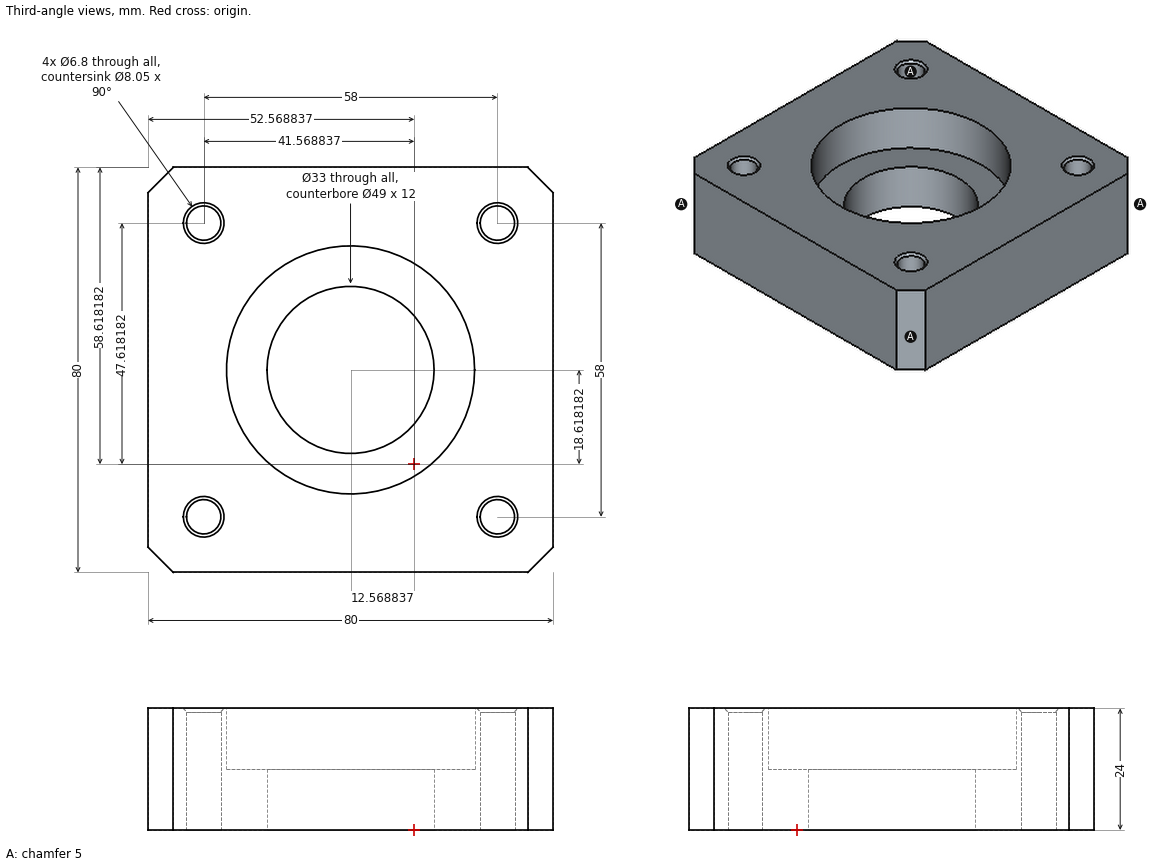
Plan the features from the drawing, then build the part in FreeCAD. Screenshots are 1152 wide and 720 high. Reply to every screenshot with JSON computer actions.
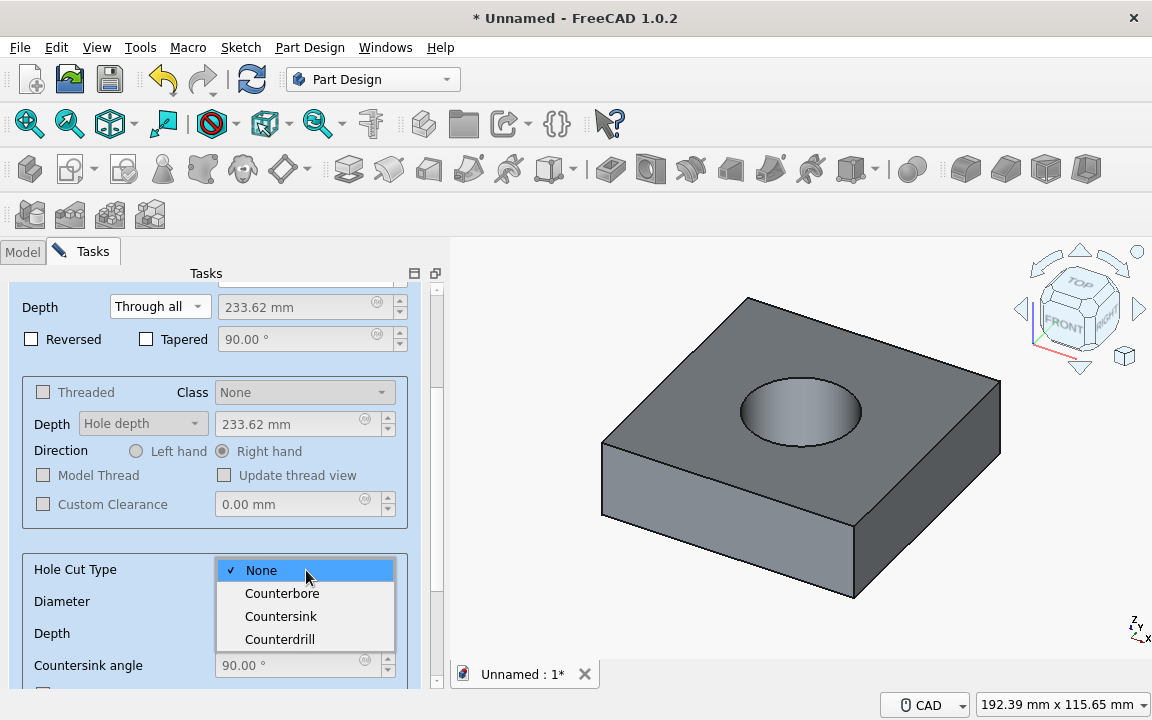
{"action": "left_click", "coordinate": [304, 594]}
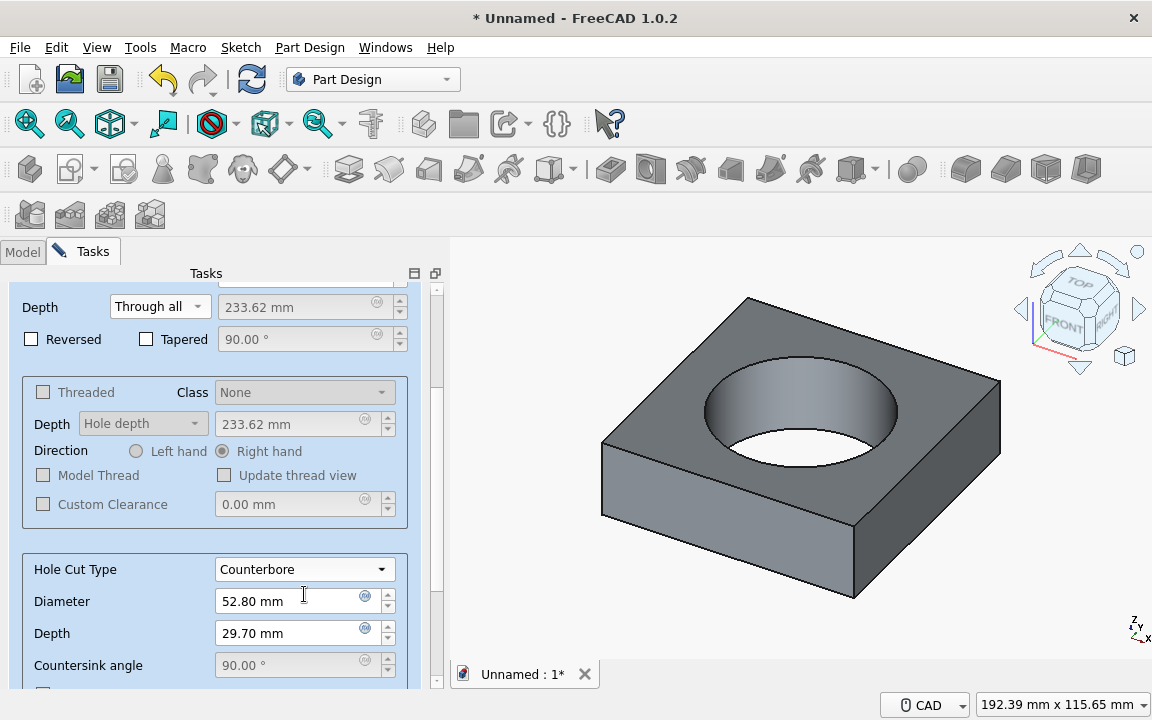
{"action": "triple_click", "coordinate": [298, 601]}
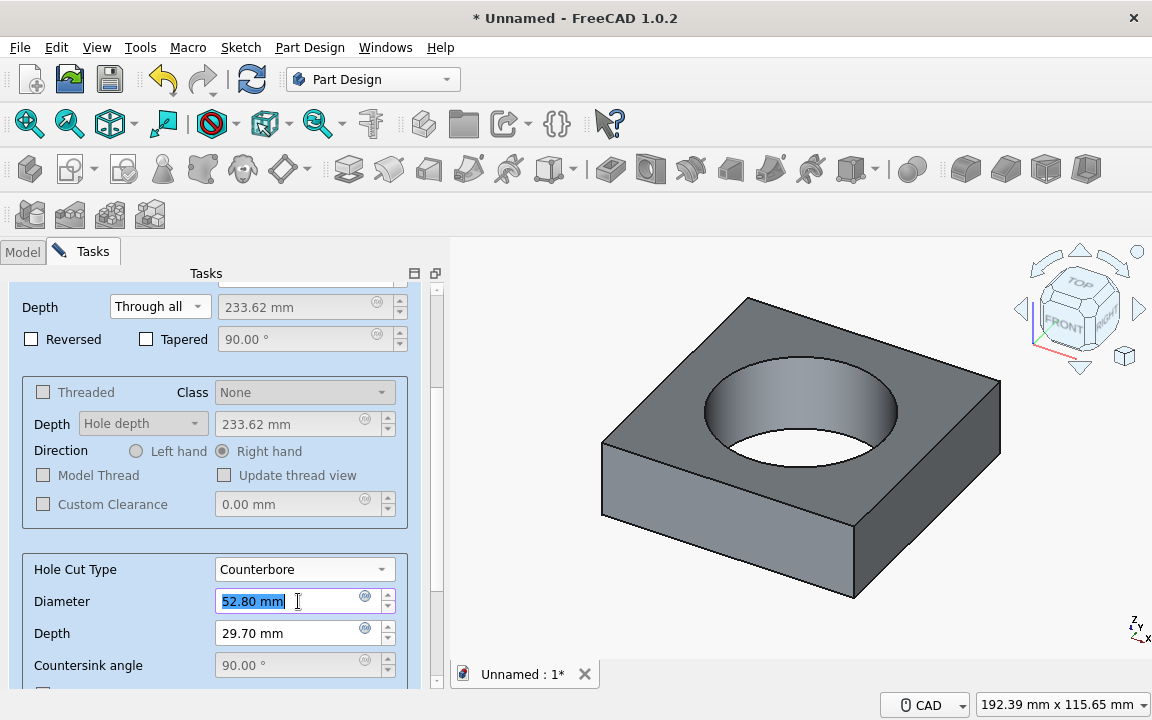
{"action": "type", "text": "49"}
{"action": "key", "text": "Tab"}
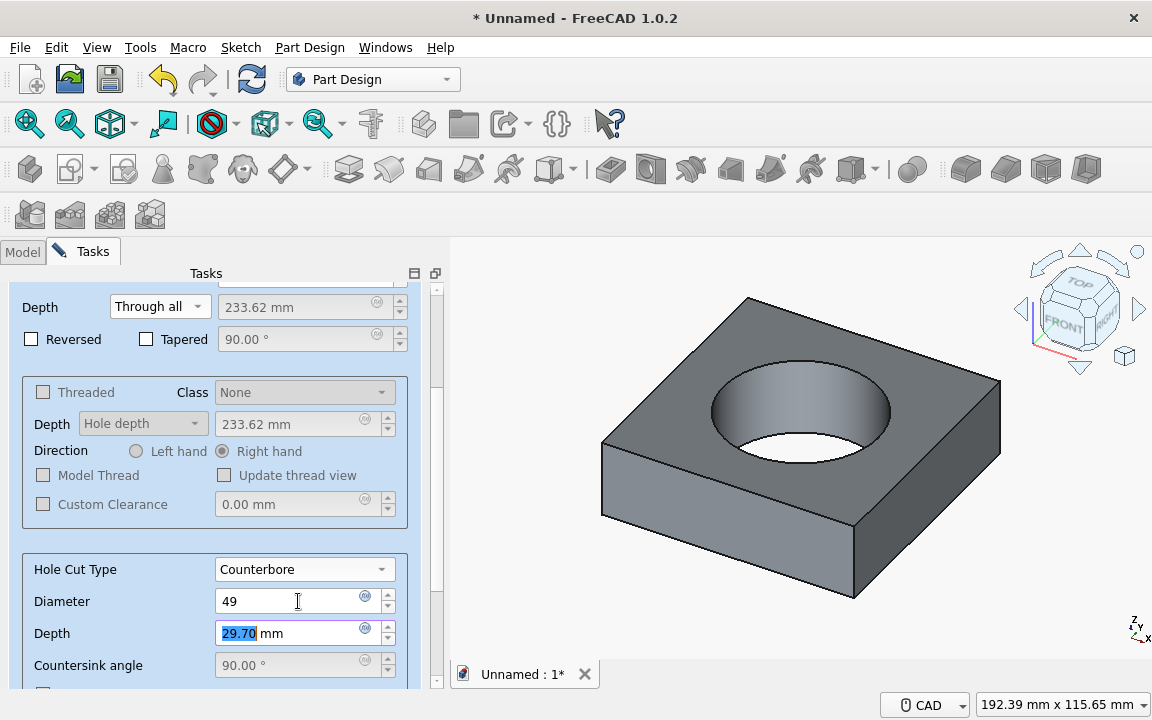
{"action": "type", "text": "12"}
{"action": "key", "text": "Tab"}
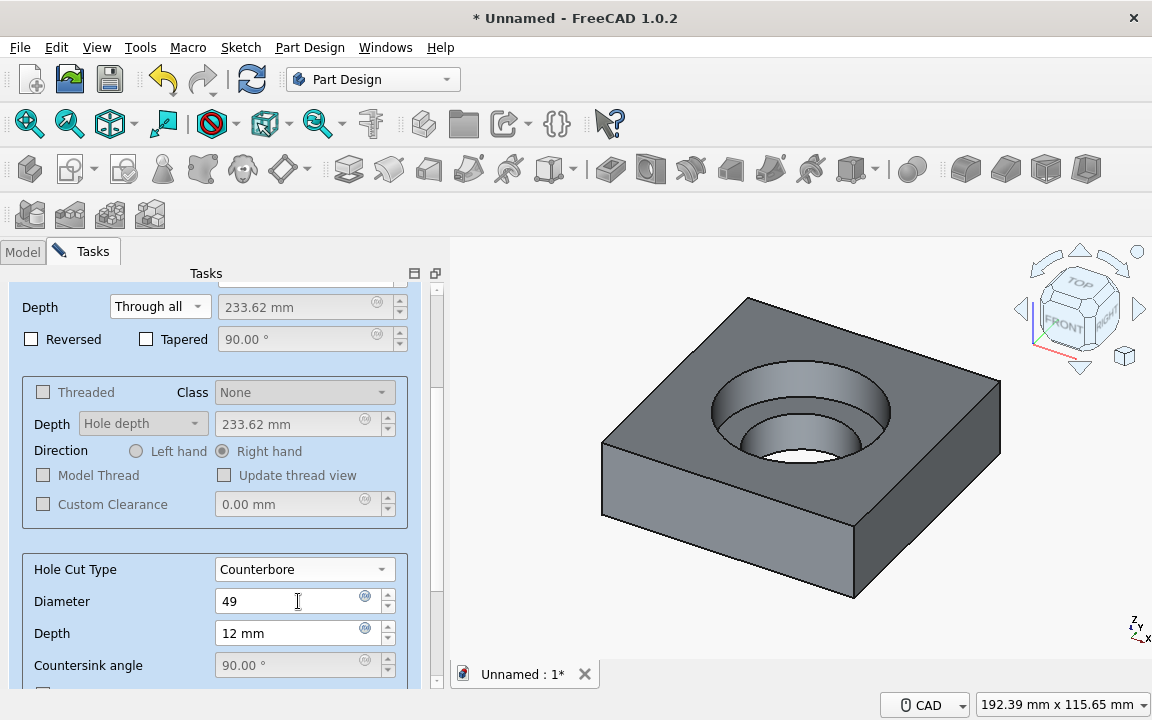
{"action": "scroll", "coordinate": [437, 486], "scroll_direction": "up", "scroll_amount": 4}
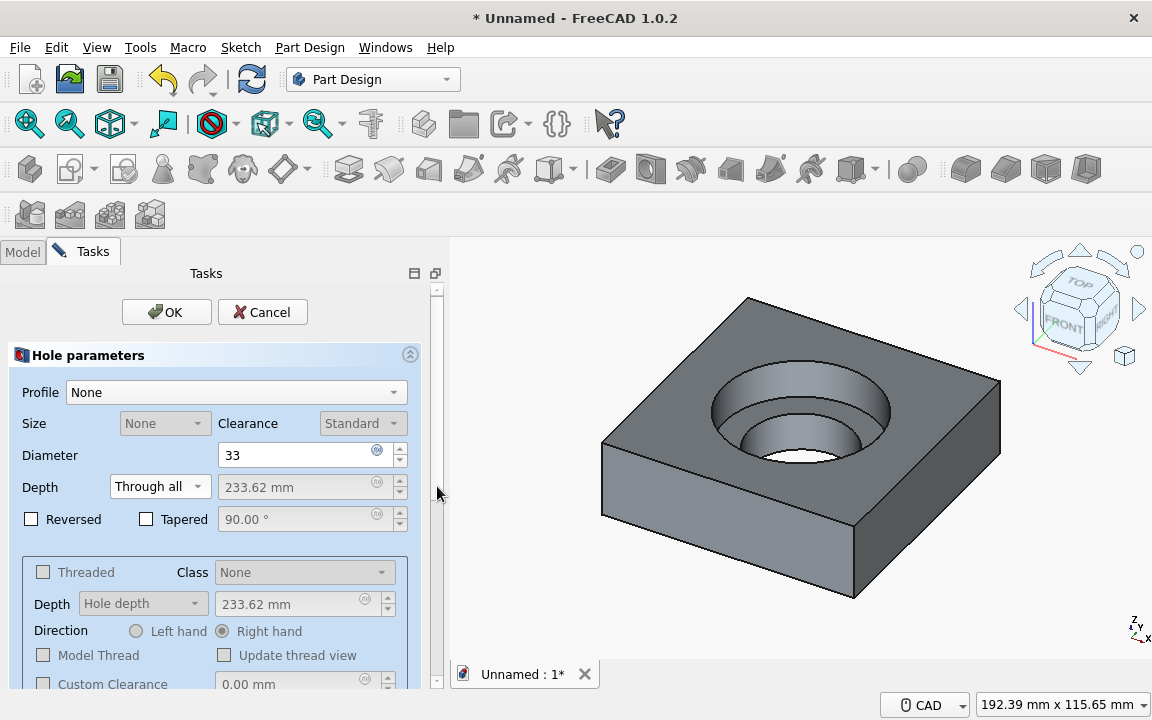
{"action": "left_click", "coordinate": [167, 312]}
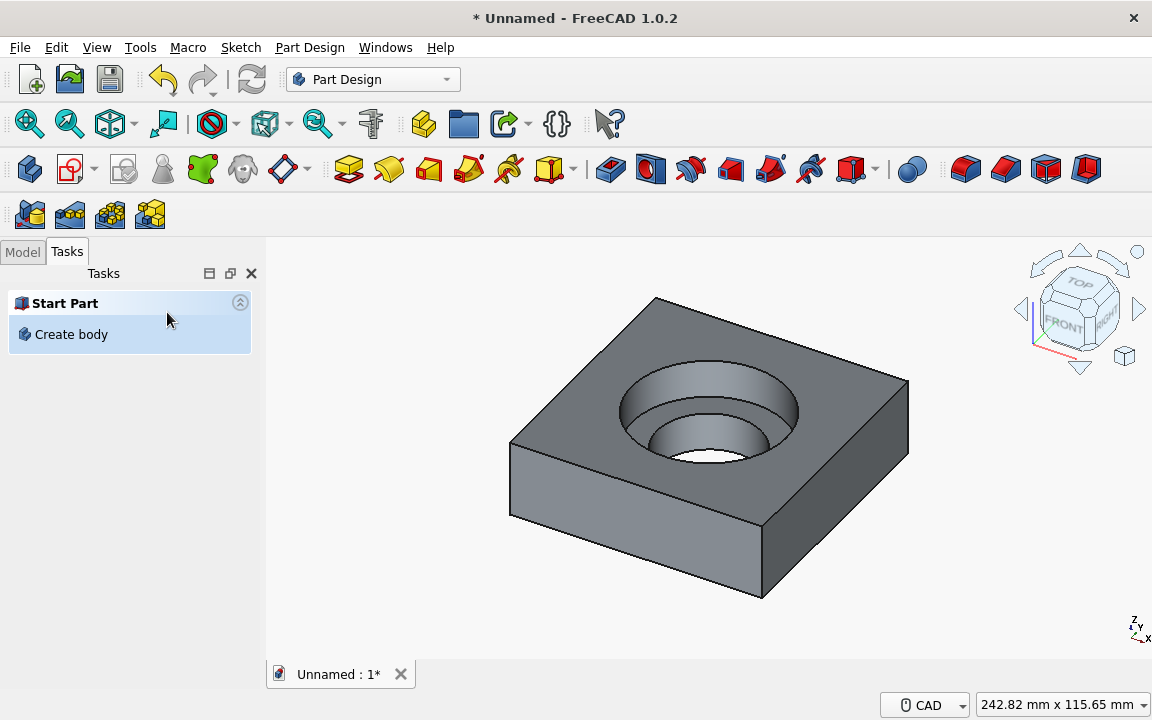
{"action": "left_click", "coordinate": [740, 476]}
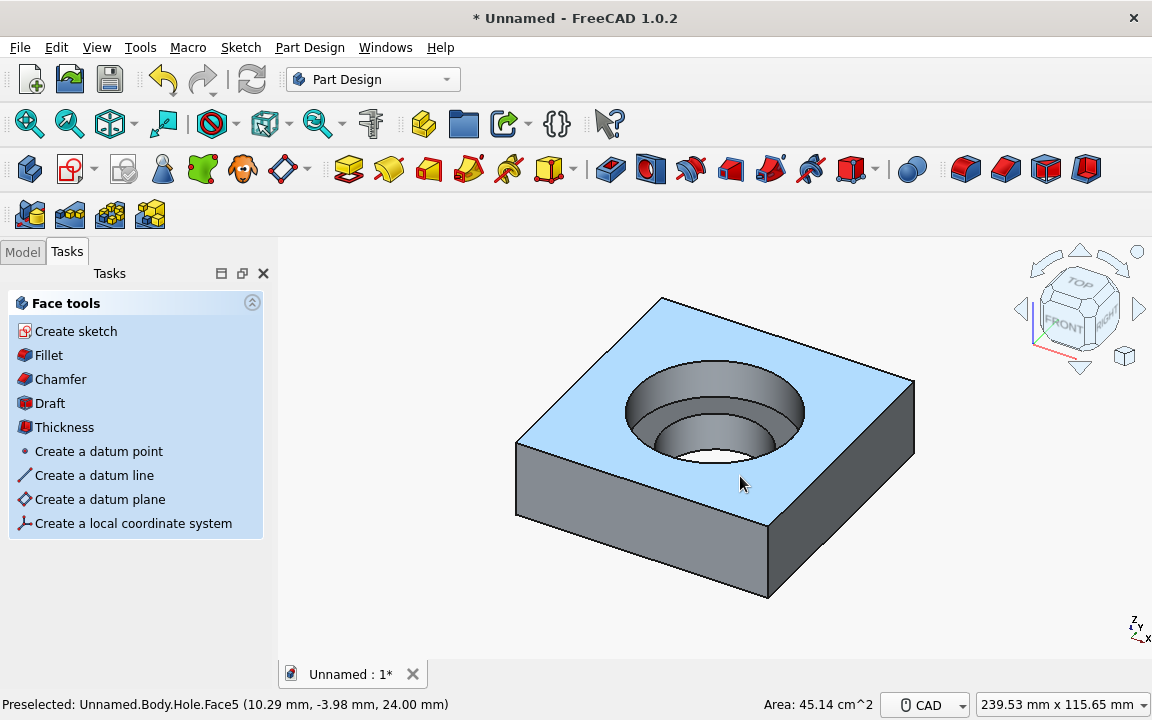
{"action": "left_click", "coordinate": [70, 170]}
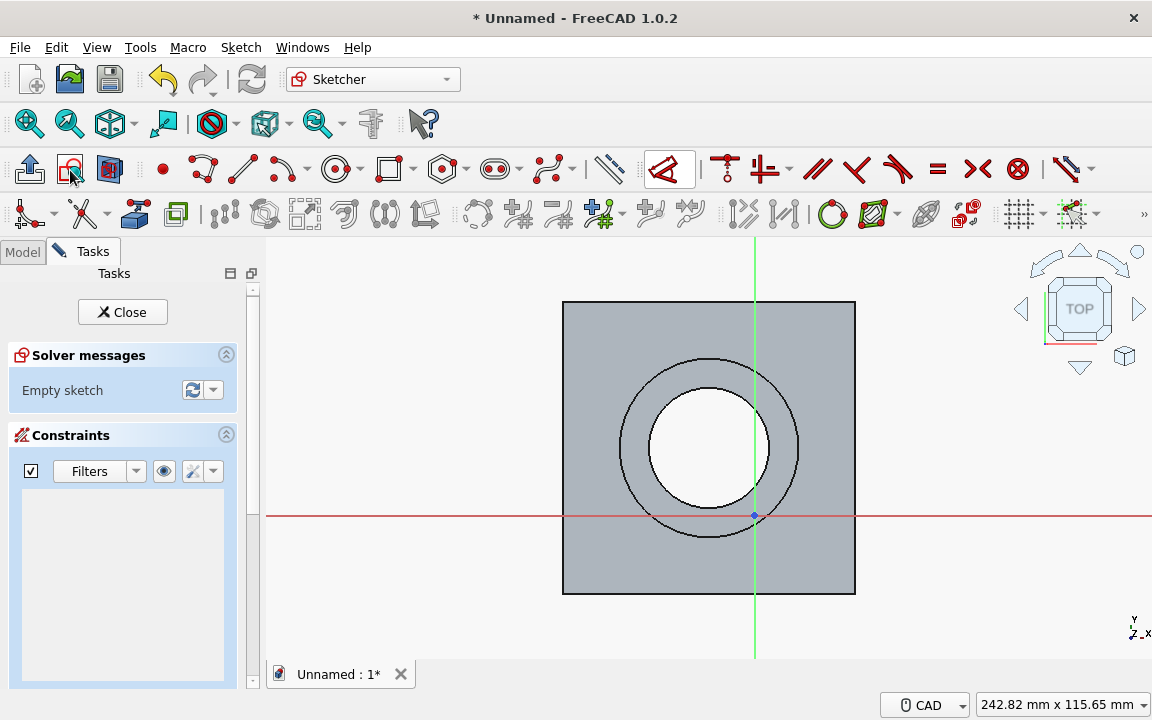
{"action": "left_click", "coordinate": [336, 170]}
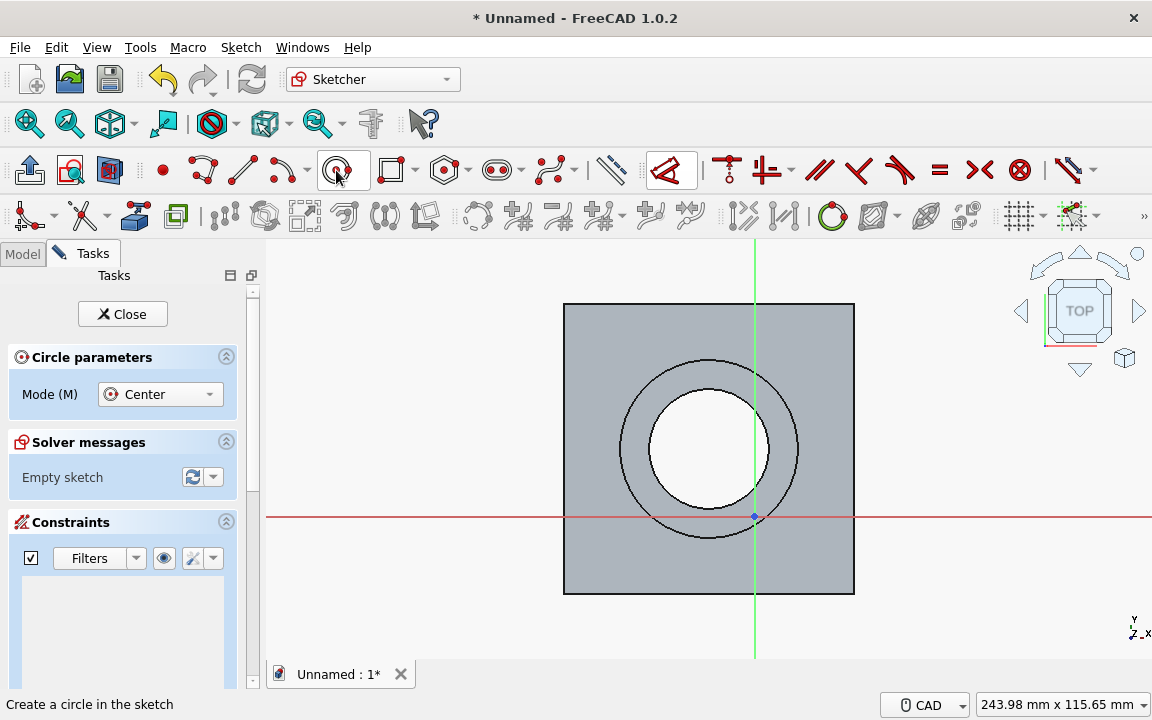
{"action": "scroll", "coordinate": [604, 344], "scroll_direction": "up", "scroll_amount": 4}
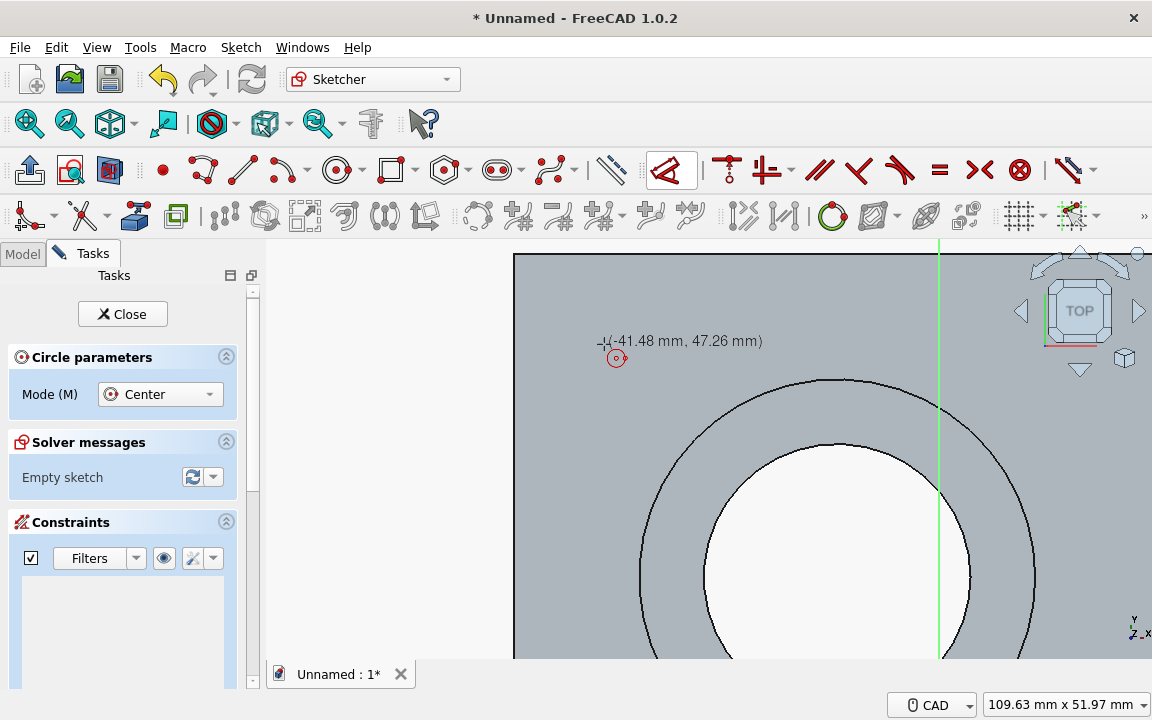
{"action": "left_click", "coordinate": [603, 343]}
{"action": "left_click", "coordinate": [622, 324]}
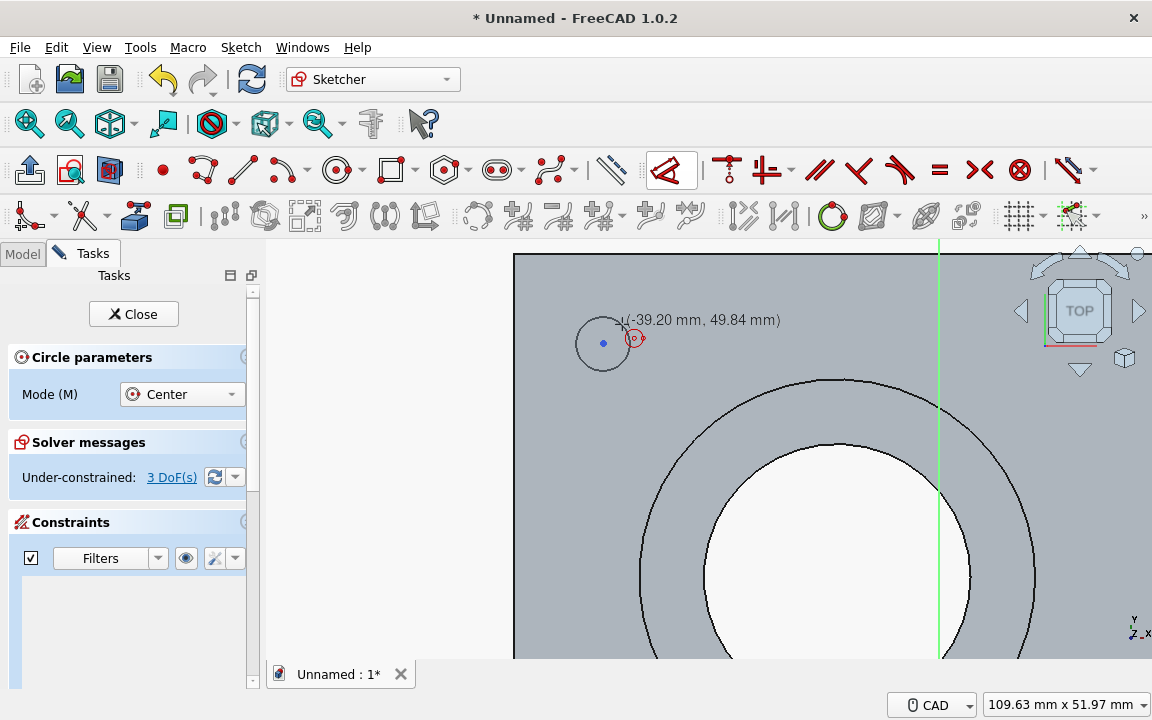
{"action": "scroll", "coordinate": [480, 344], "scroll_direction": "down", "scroll_amount": 4}